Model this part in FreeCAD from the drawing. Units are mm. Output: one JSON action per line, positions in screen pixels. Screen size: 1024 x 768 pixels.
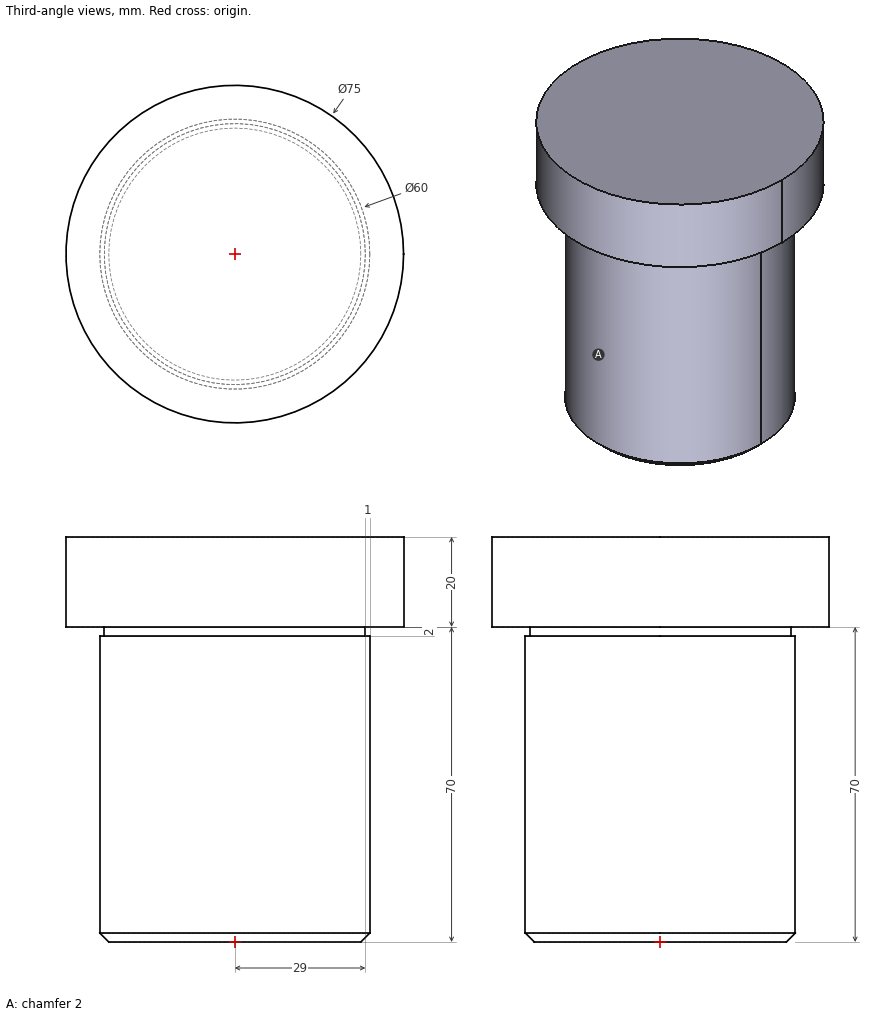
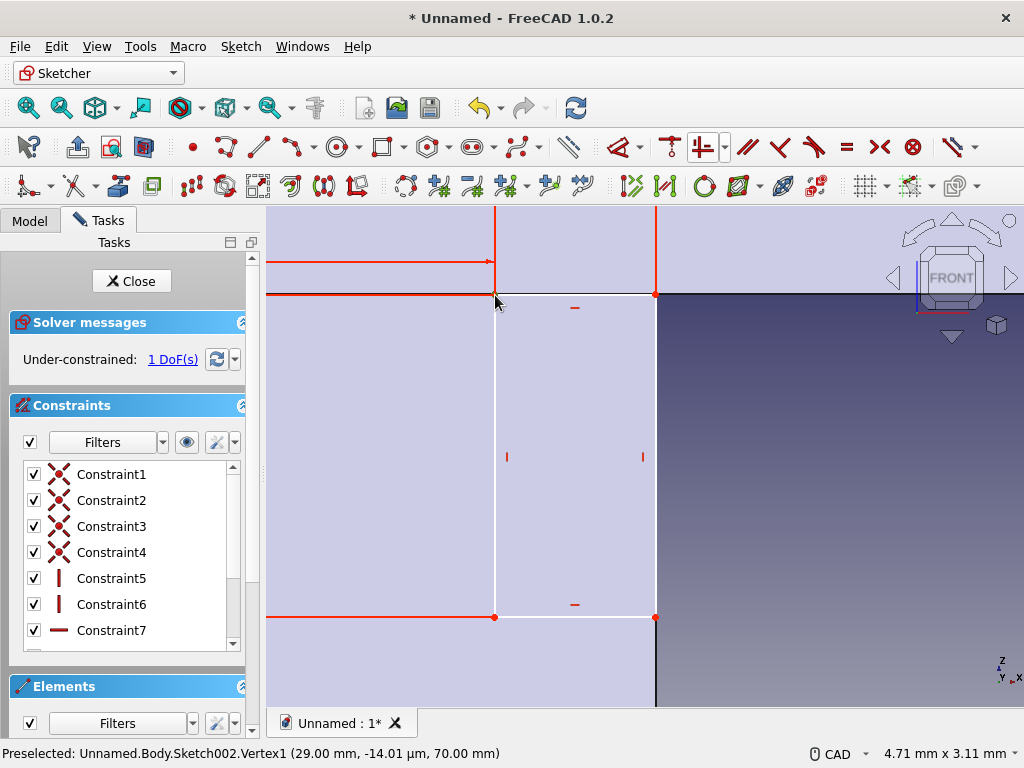
{"action": "key", "text": "i"}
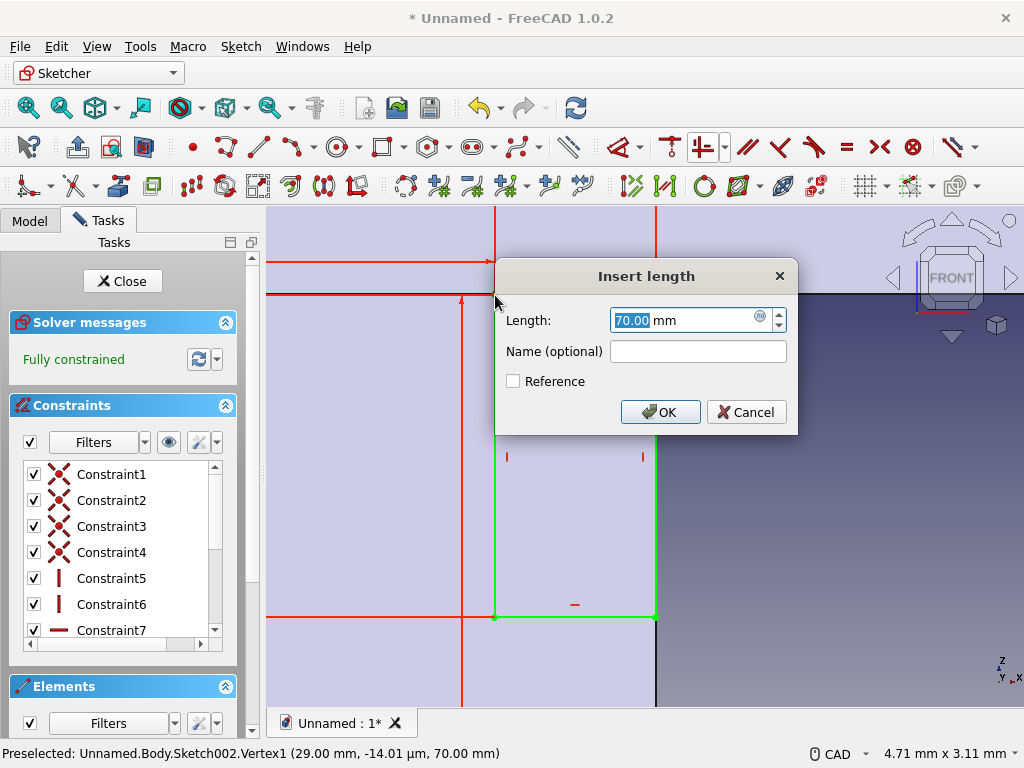
{"action": "type", "text": "70"}
{"action": "key", "text": "Return"}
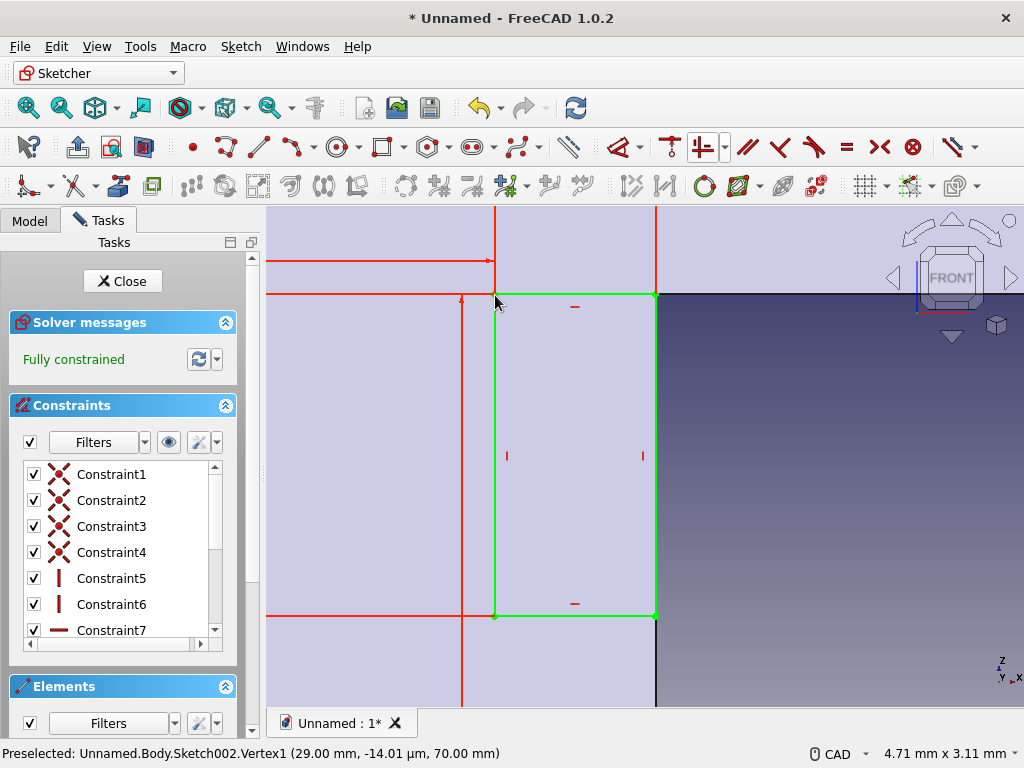
{"action": "left_click", "coordinate": [123, 281]}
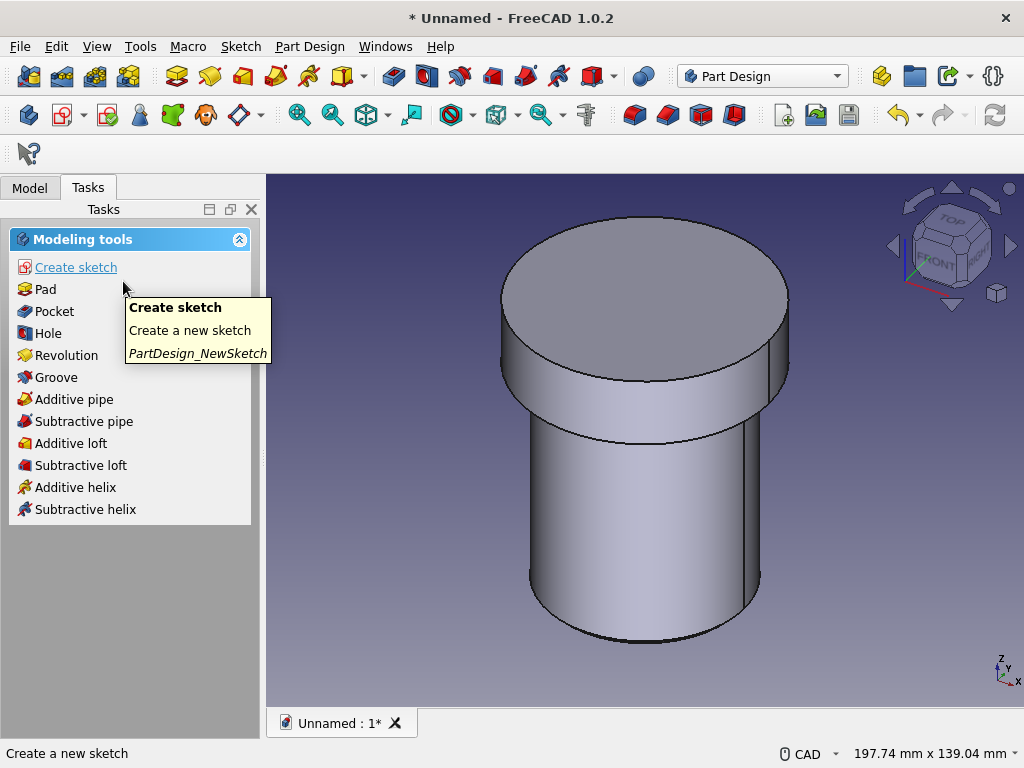
{"action": "left_click", "coordinate": [460, 76]}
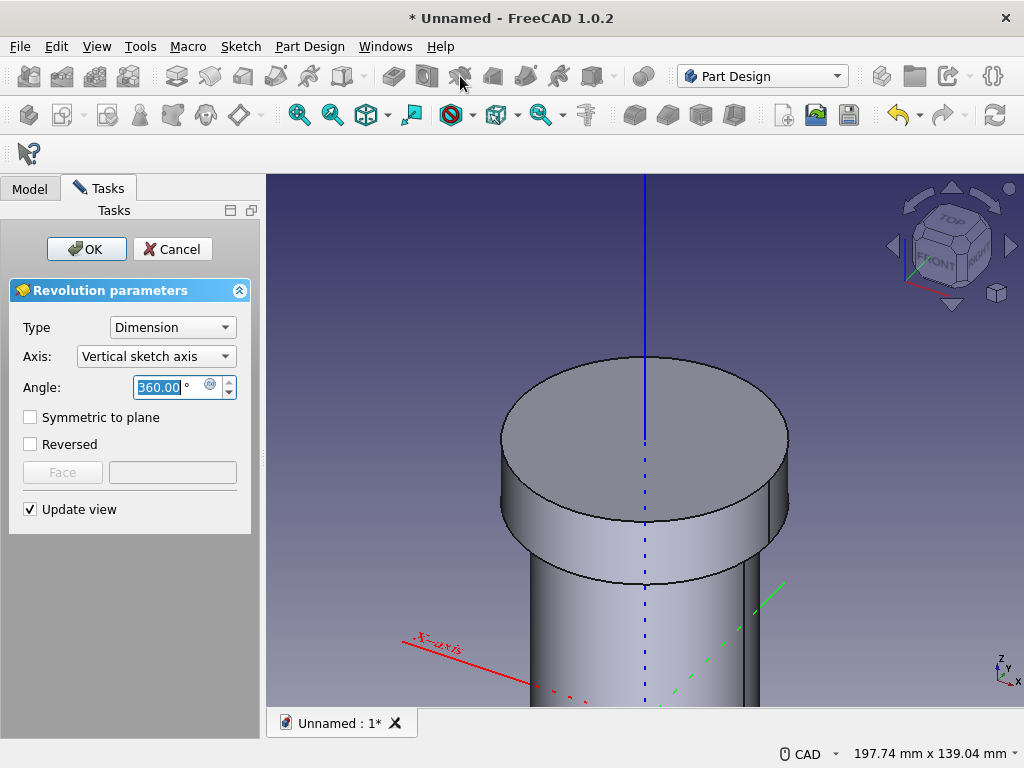
{"action": "left_click", "coordinate": [87, 249]}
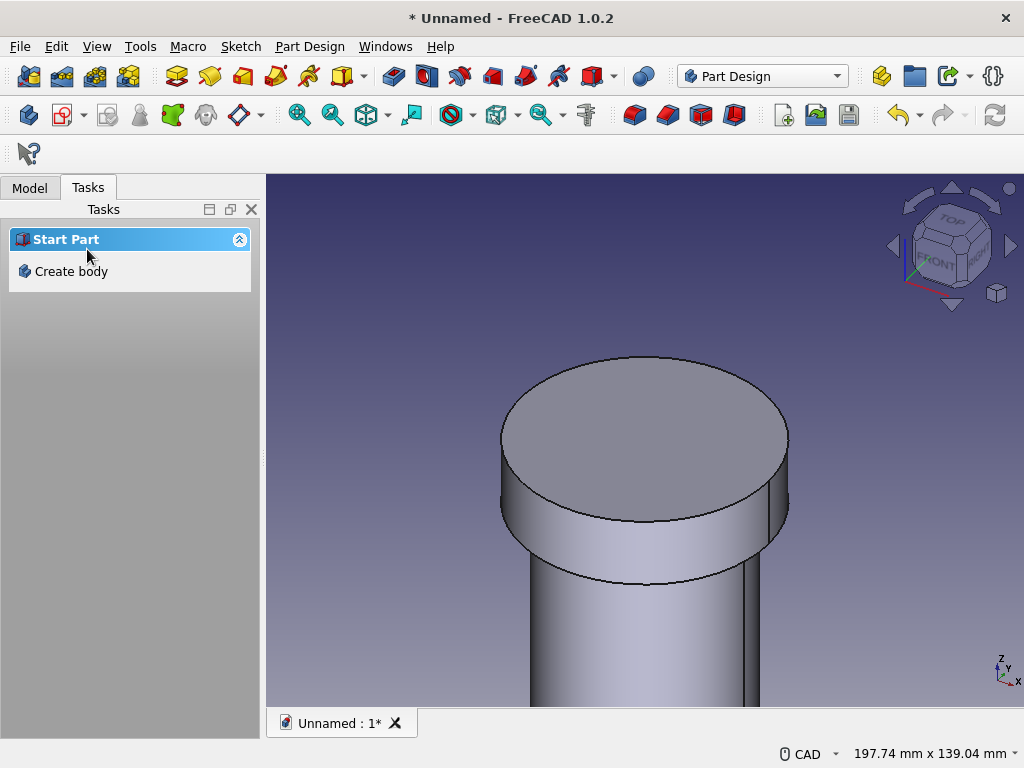
{"action": "key", "text": "0"}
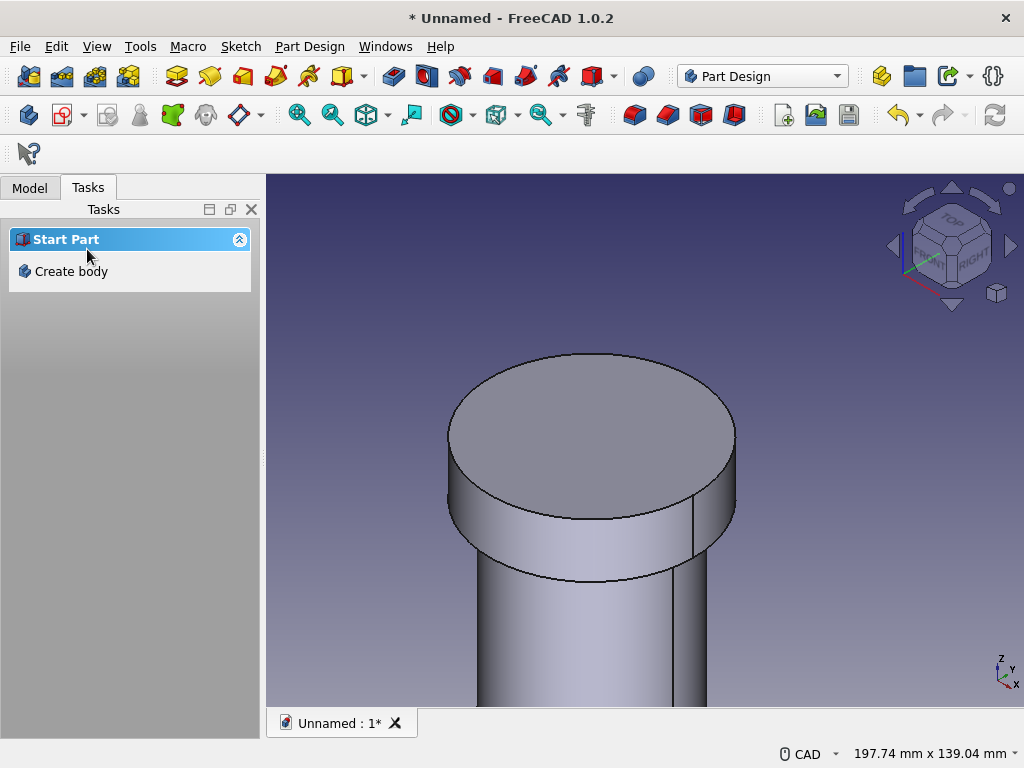
{"action": "key", "text": "v f"}